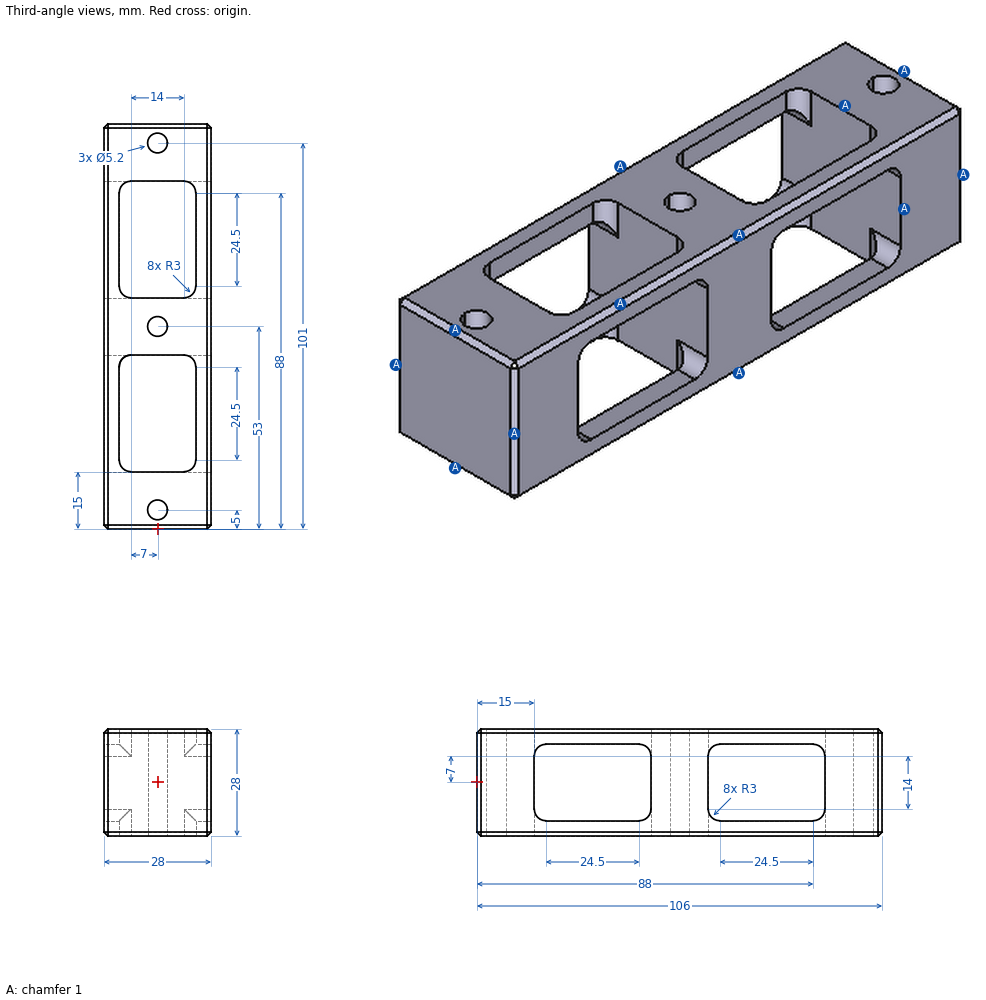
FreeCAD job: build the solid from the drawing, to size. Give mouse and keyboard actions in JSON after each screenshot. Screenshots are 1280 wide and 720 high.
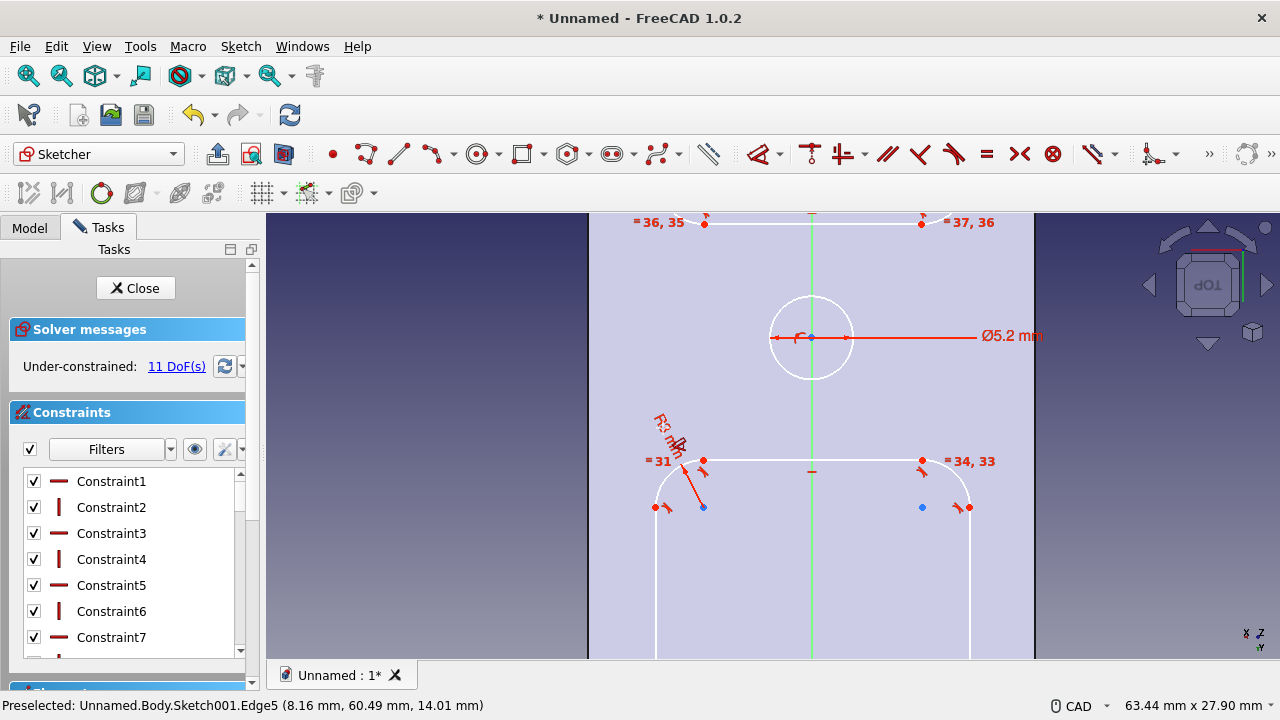
{"action": "scroll", "coordinate": [683, 460], "scroll_direction": "down", "scroll_amount": 9}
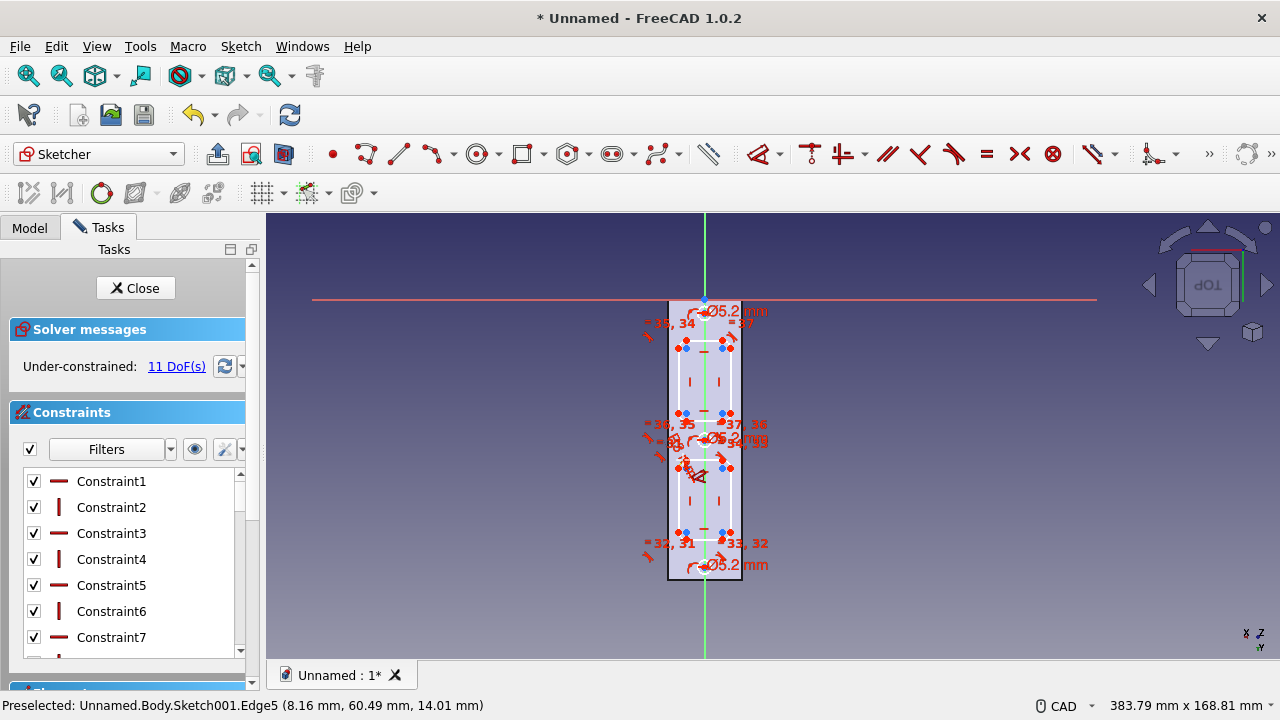
{"action": "scroll", "coordinate": [705, 313], "scroll_direction": "up", "scroll_amount": 6}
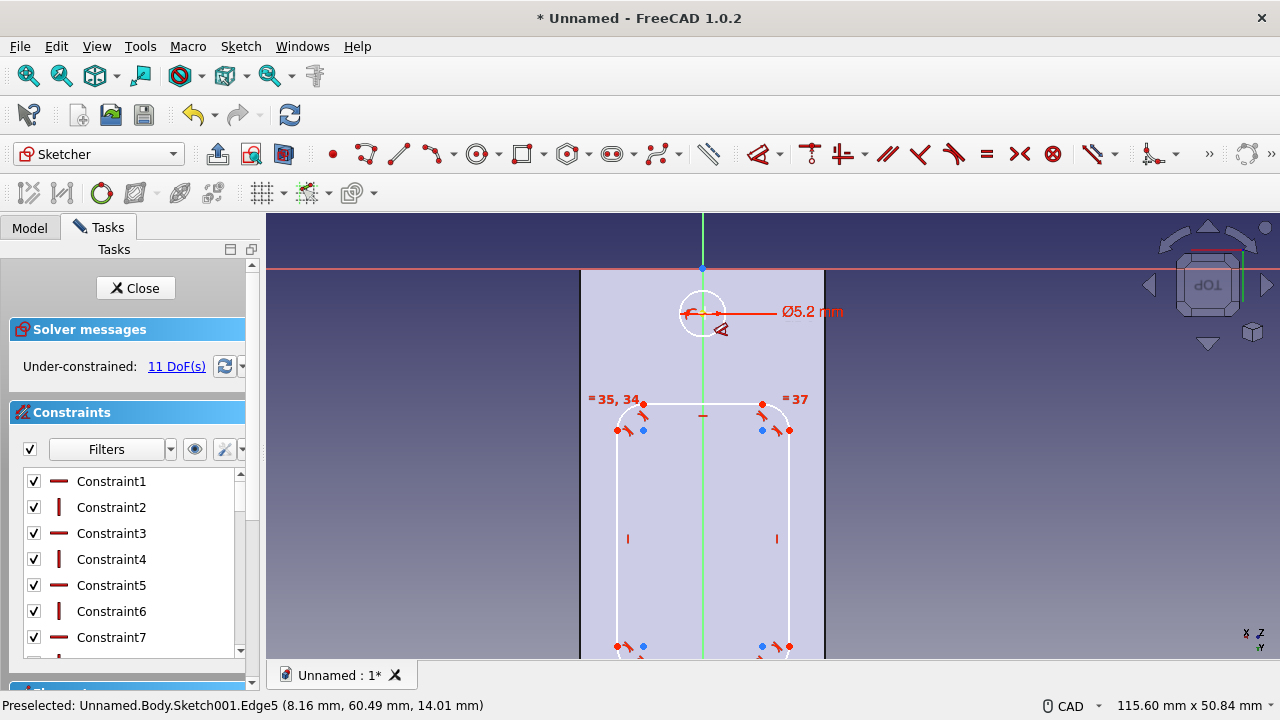
{"action": "left_click", "coordinate": [703, 314]}
{"action": "left_click", "coordinate": [737, 291]}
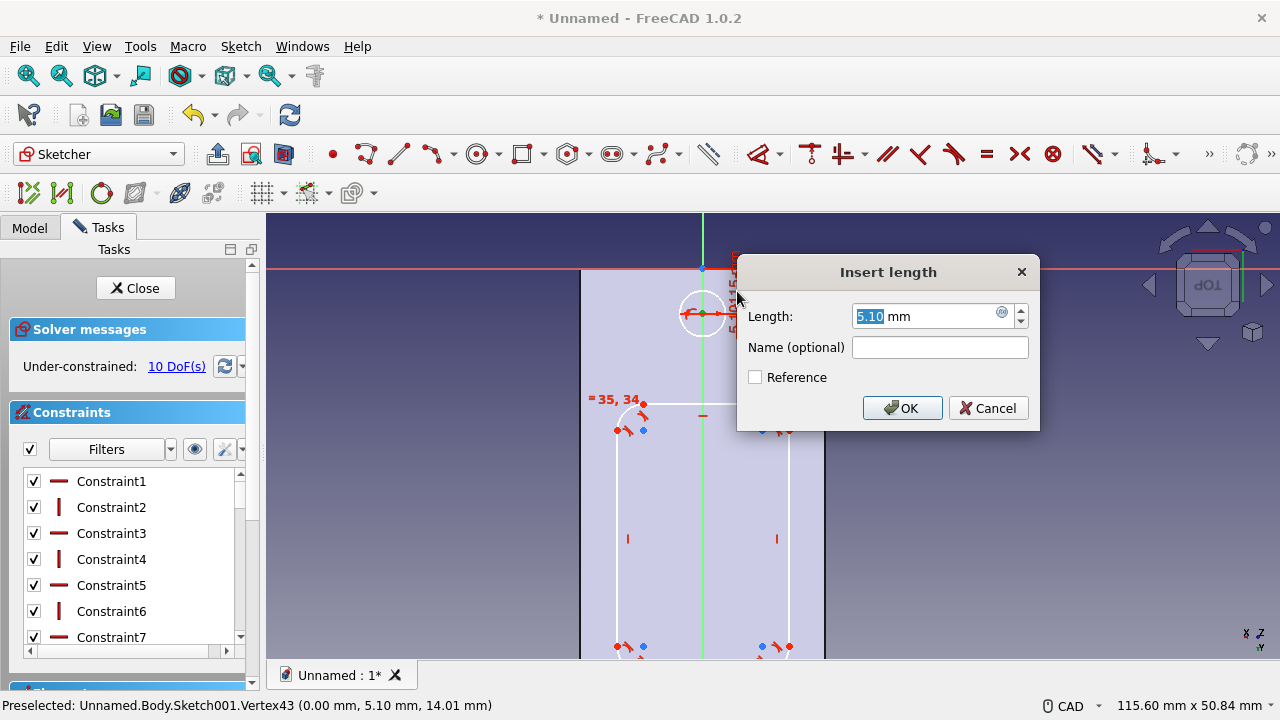
{"action": "type", "text": "5"}
{"action": "key", "text": "Return"}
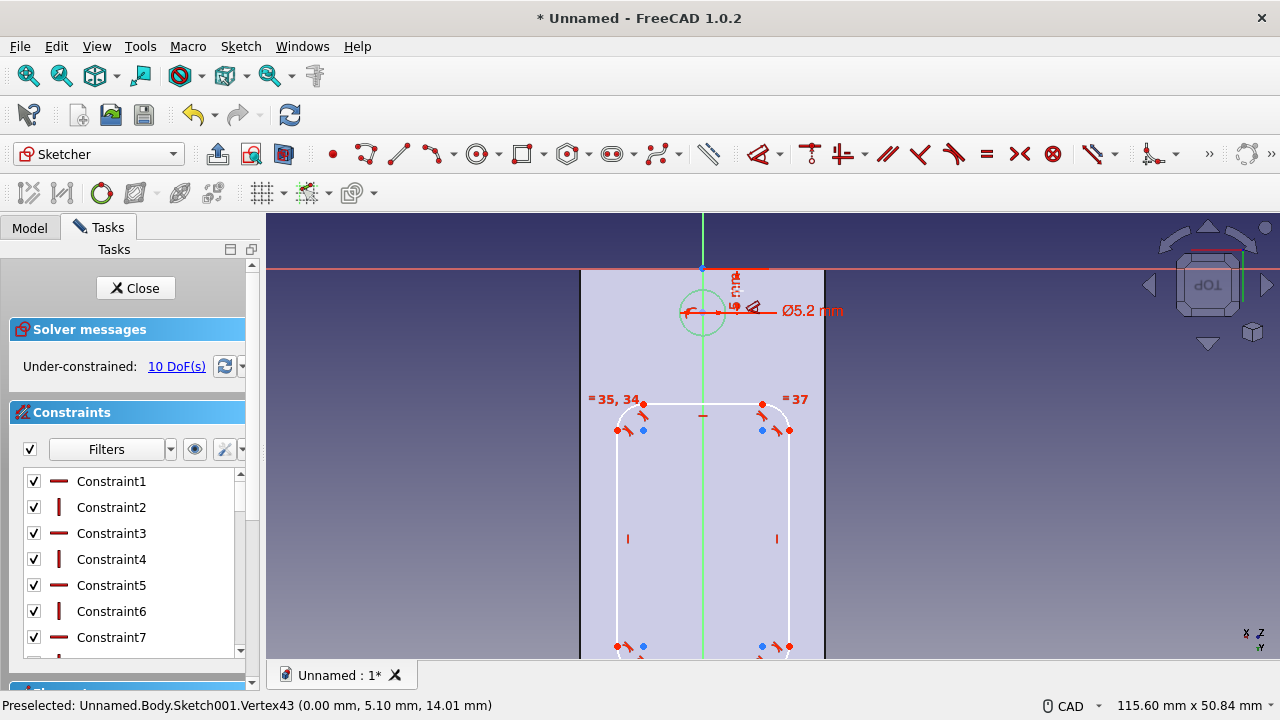
{"action": "scroll", "coordinate": [705, 312], "scroll_direction": "down", "scroll_amount": 6}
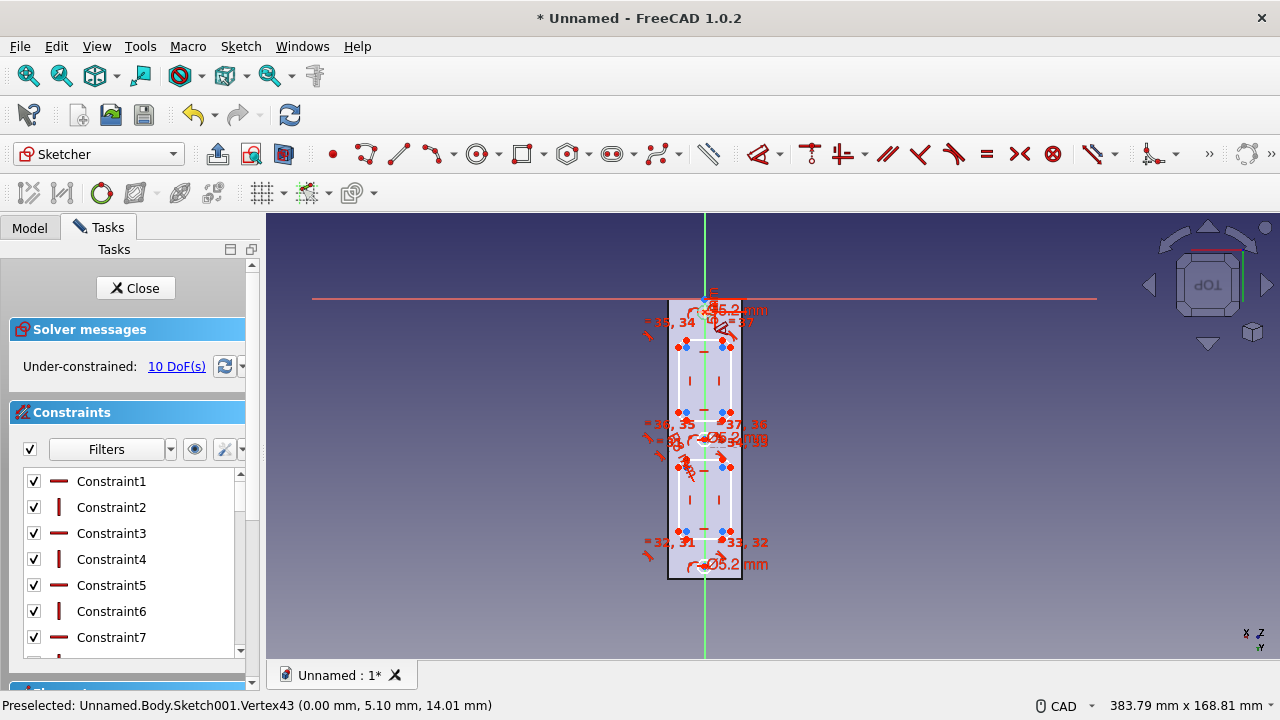
{"action": "scroll", "coordinate": [712, 460], "scroll_direction": "up", "scroll_amount": 4}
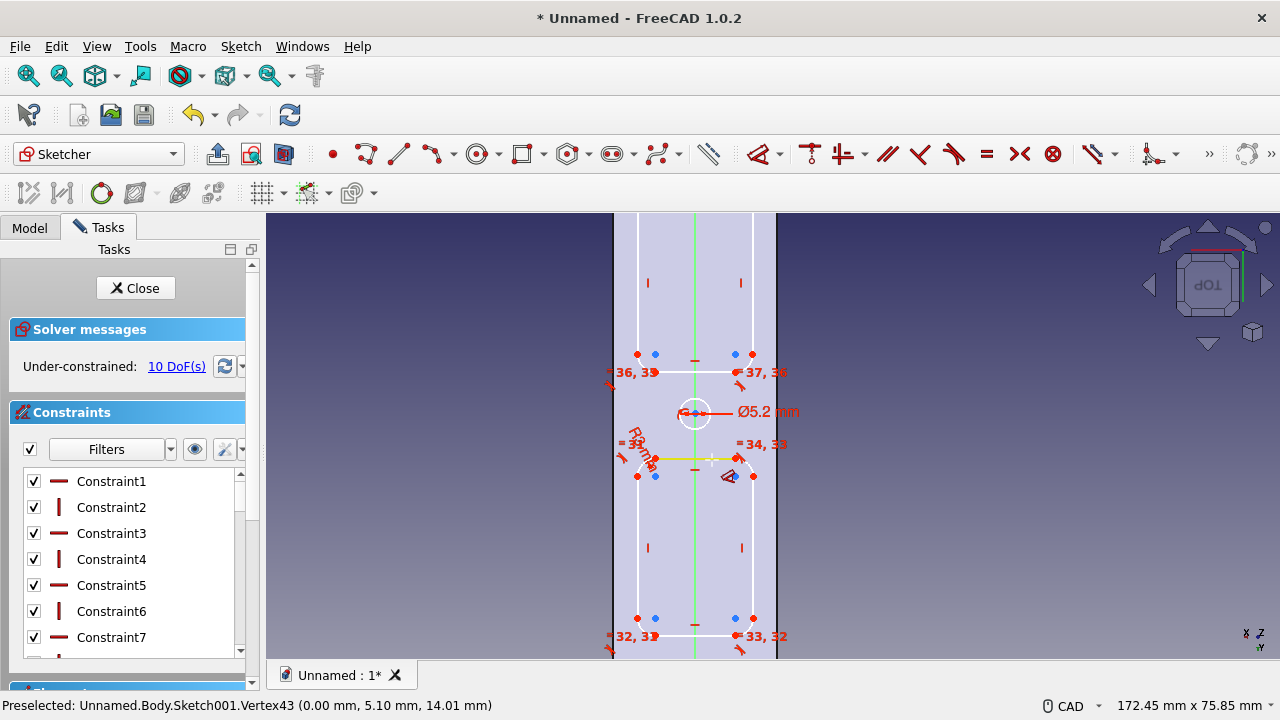
{"action": "left_click", "coordinate": [712, 459]}
{"action": "left_click", "coordinate": [677, 493]}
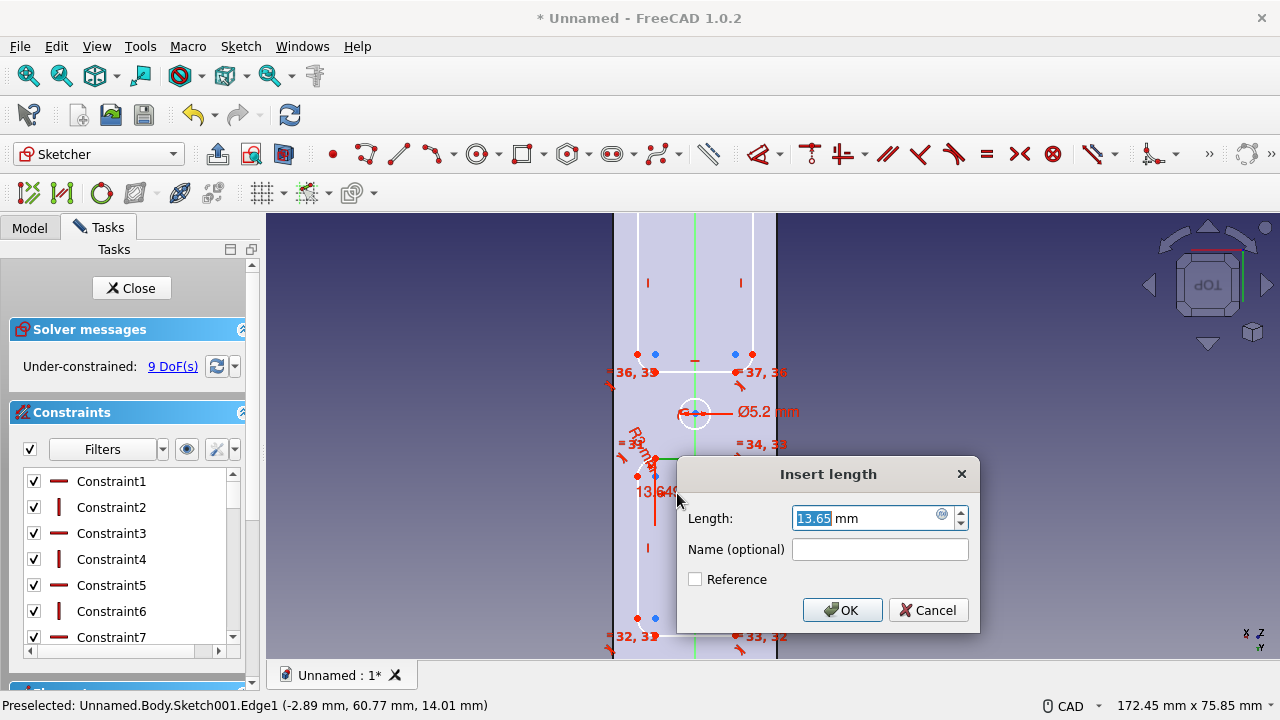
{"action": "type", "text": "14"}
{"action": "key", "text": "Return"}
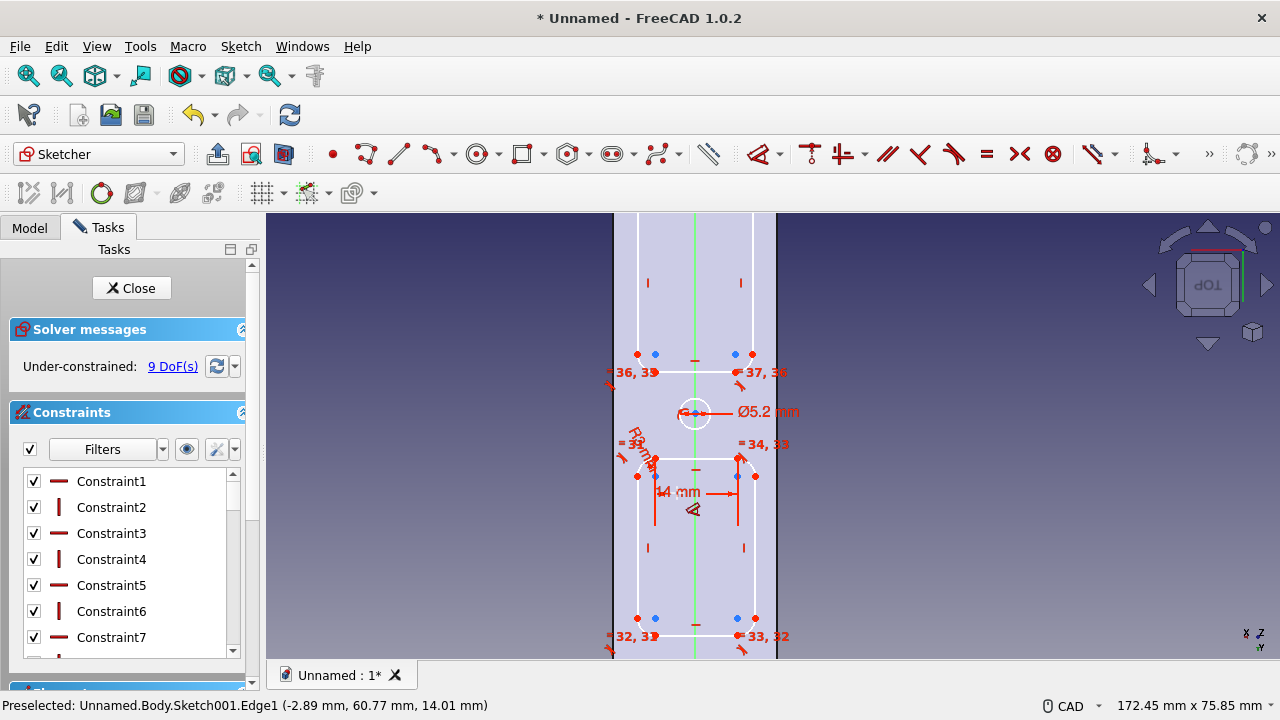
{"action": "scroll", "coordinate": [712, 460], "scroll_direction": "down", "scroll_amount": 4}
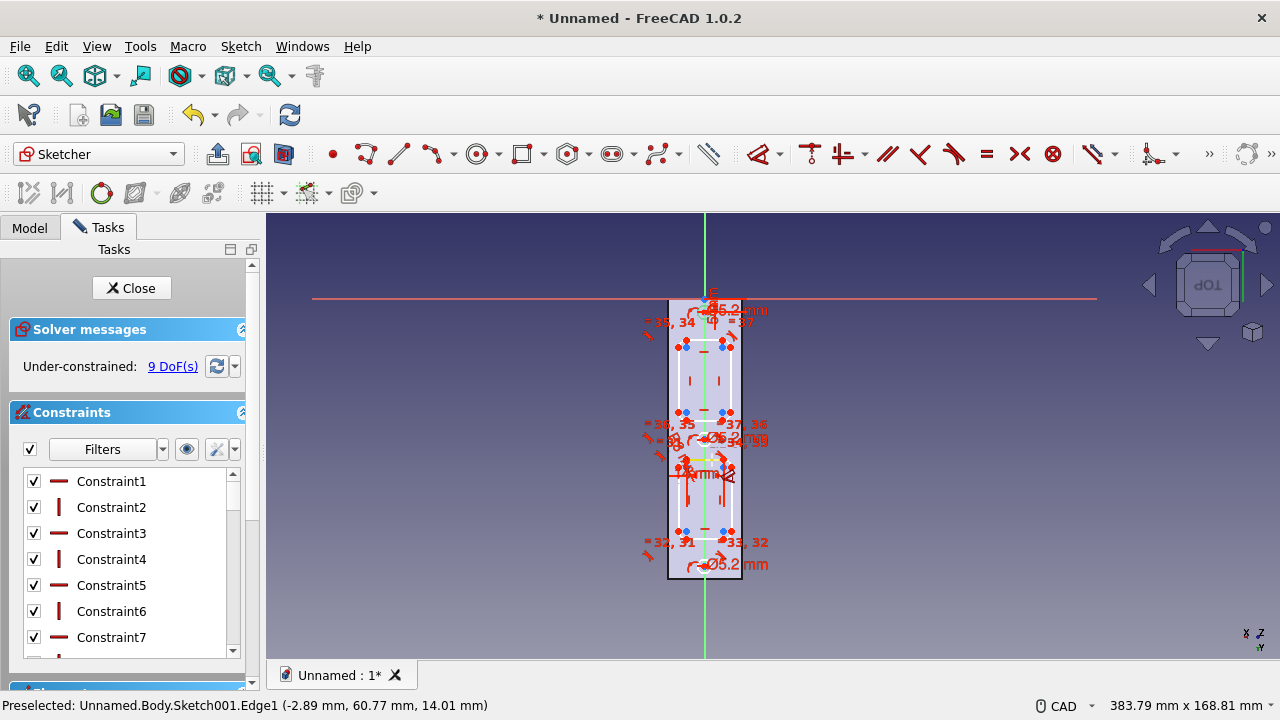
{"action": "scroll", "coordinate": [712, 340], "scroll_direction": "up", "scroll_amount": 4}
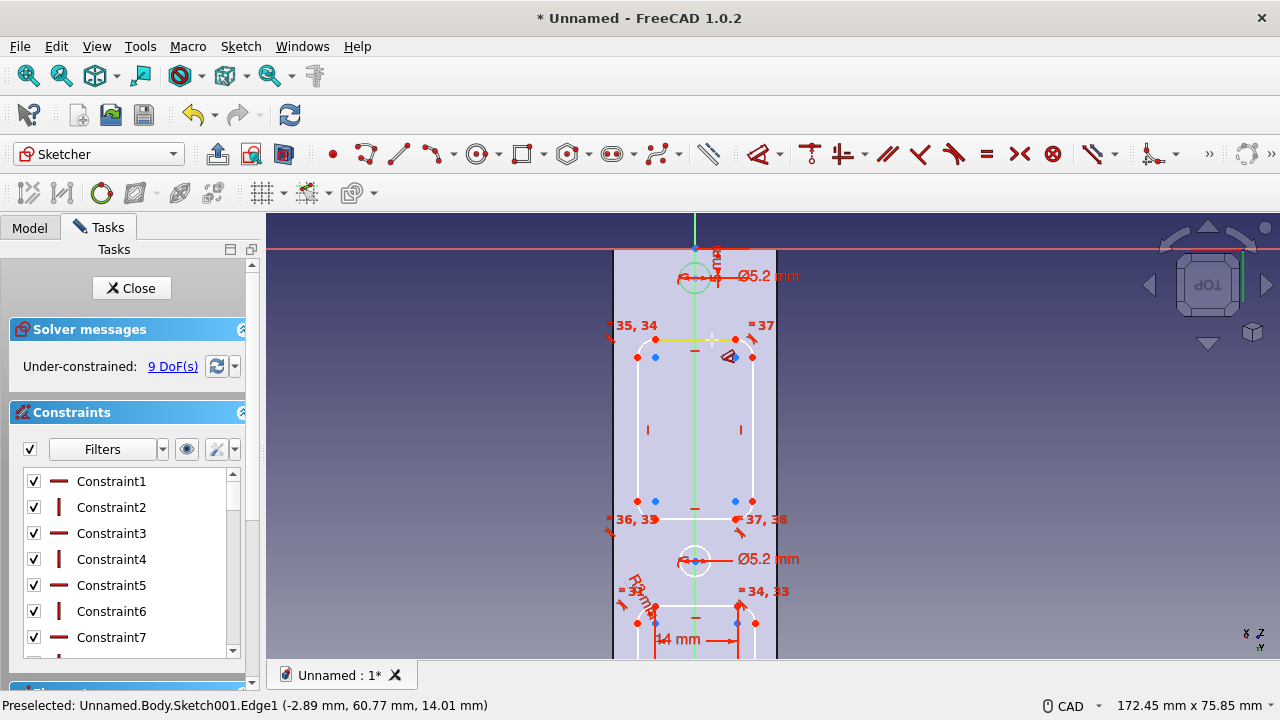
{"action": "left_click", "coordinate": [711, 340]}
{"action": "left_click", "coordinate": [677, 306]}